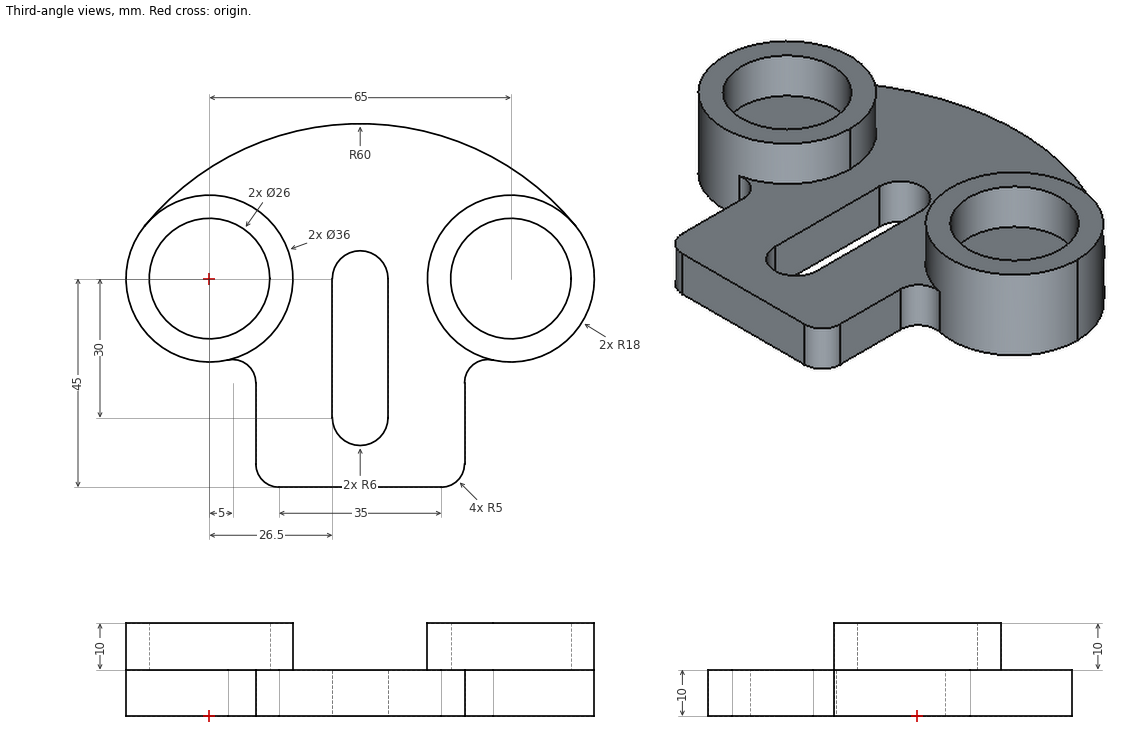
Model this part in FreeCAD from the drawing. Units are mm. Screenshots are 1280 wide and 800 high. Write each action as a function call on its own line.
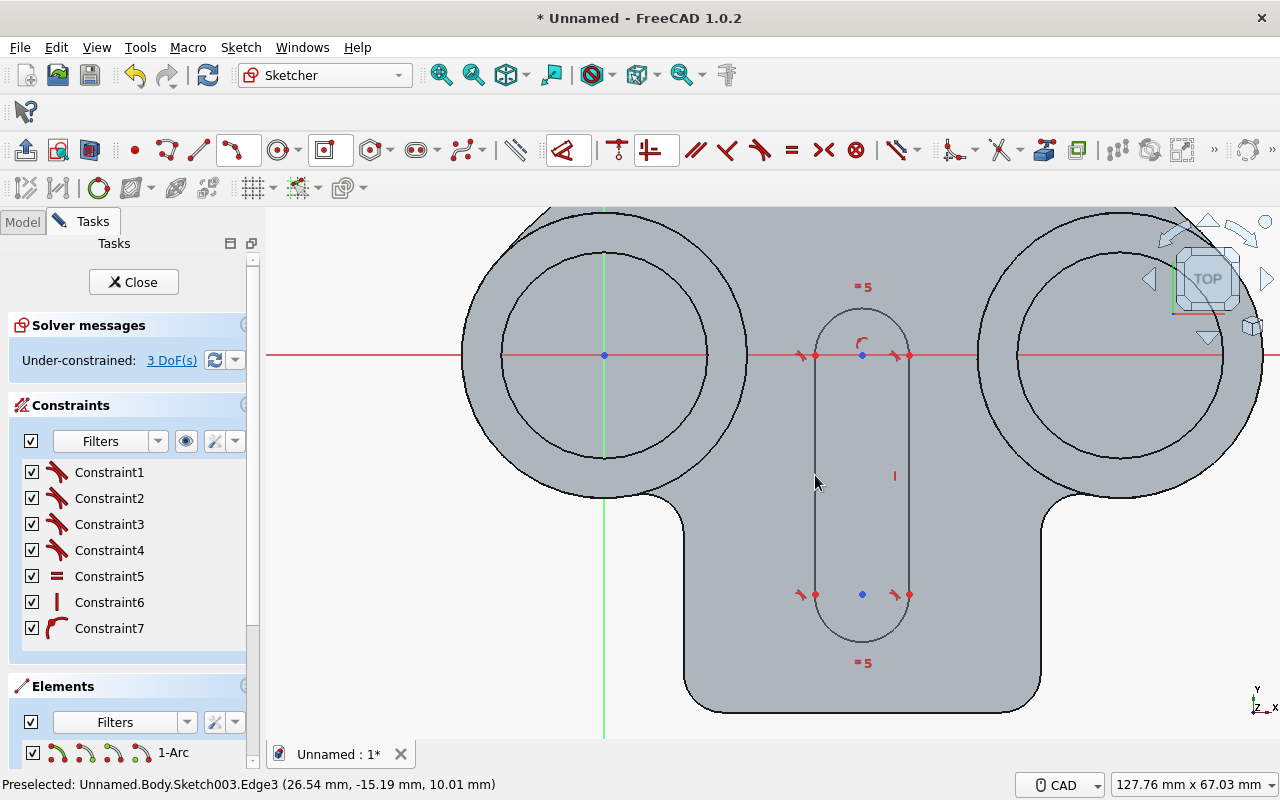
click(834, 633)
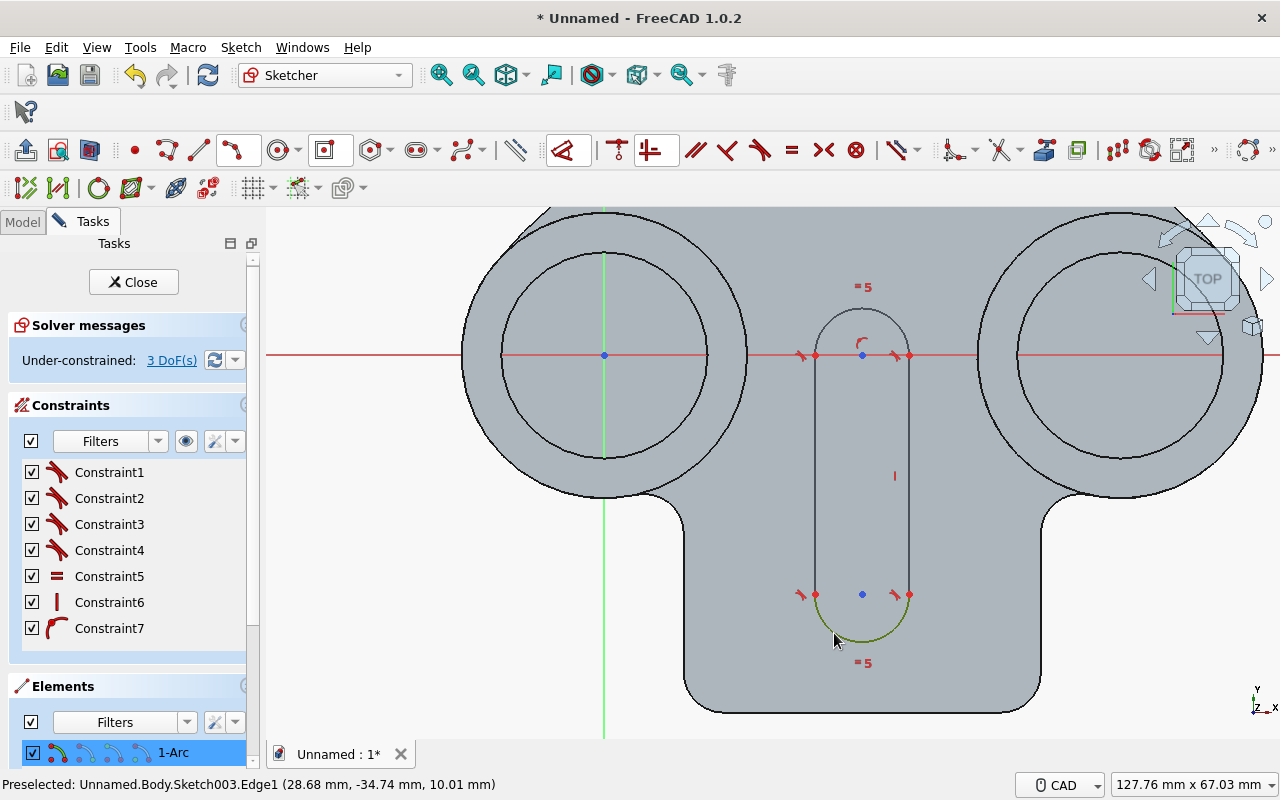
key(k)
key(r)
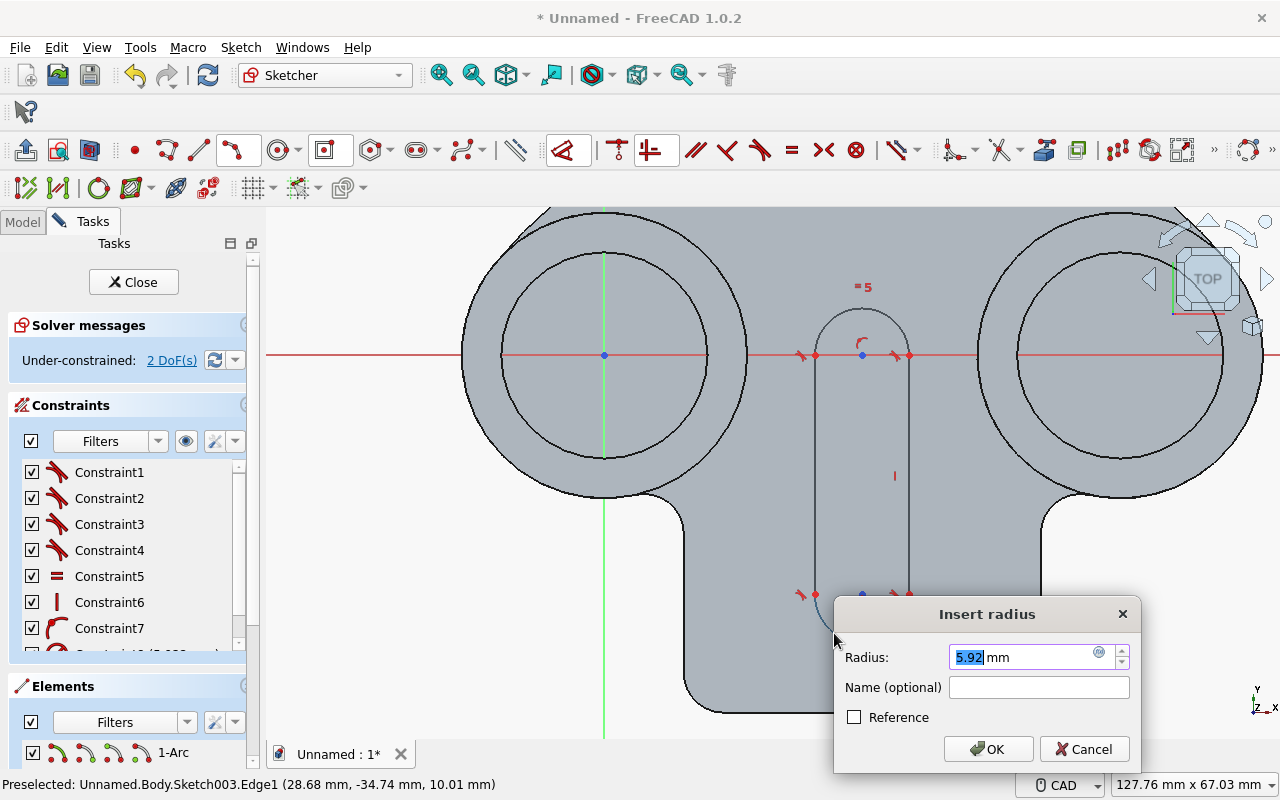
text(6)
key(Return)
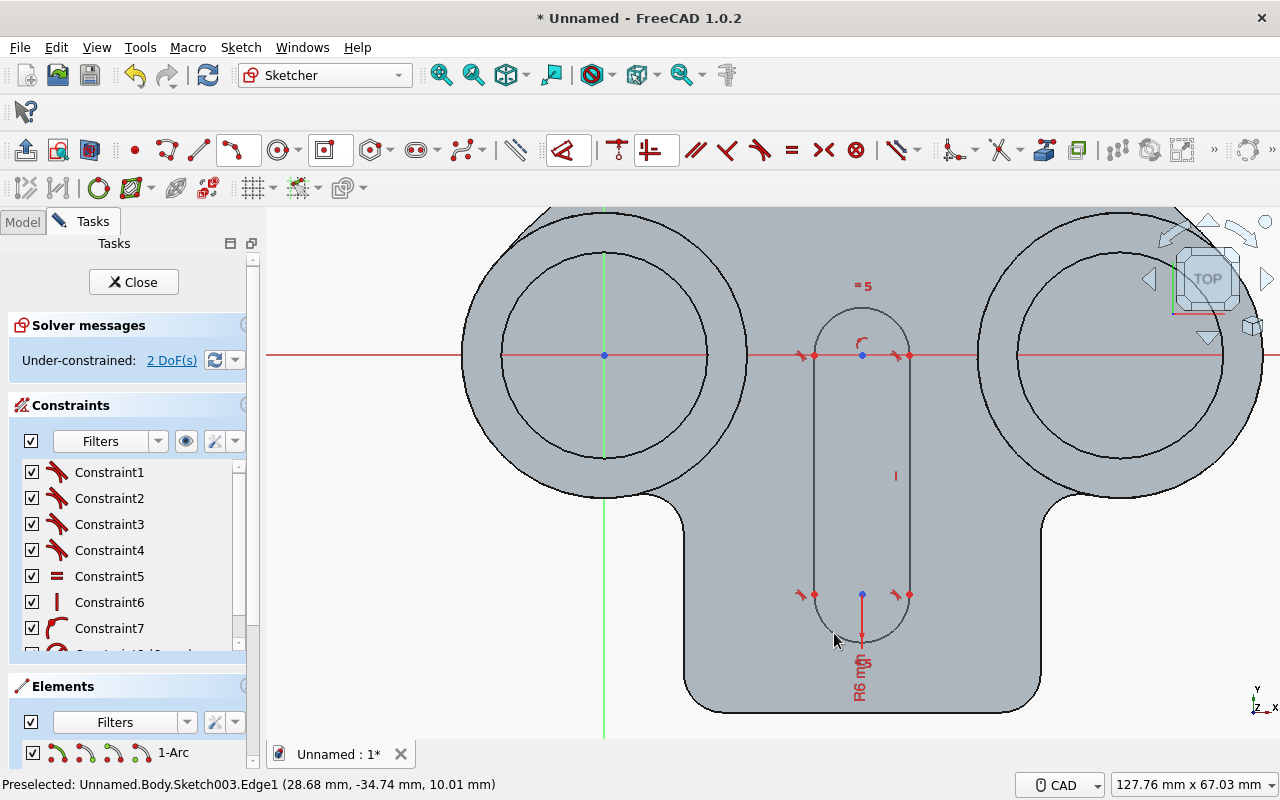
click(814, 523)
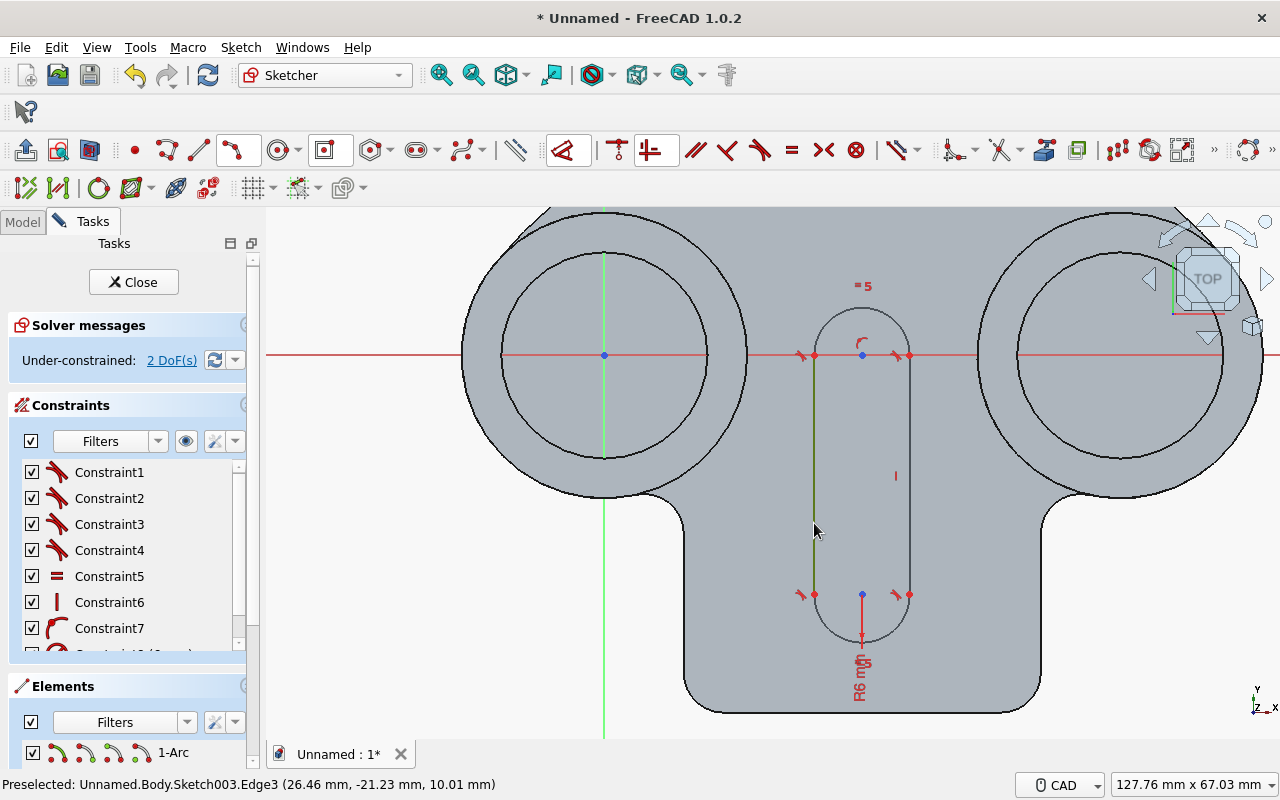
click(586, 150)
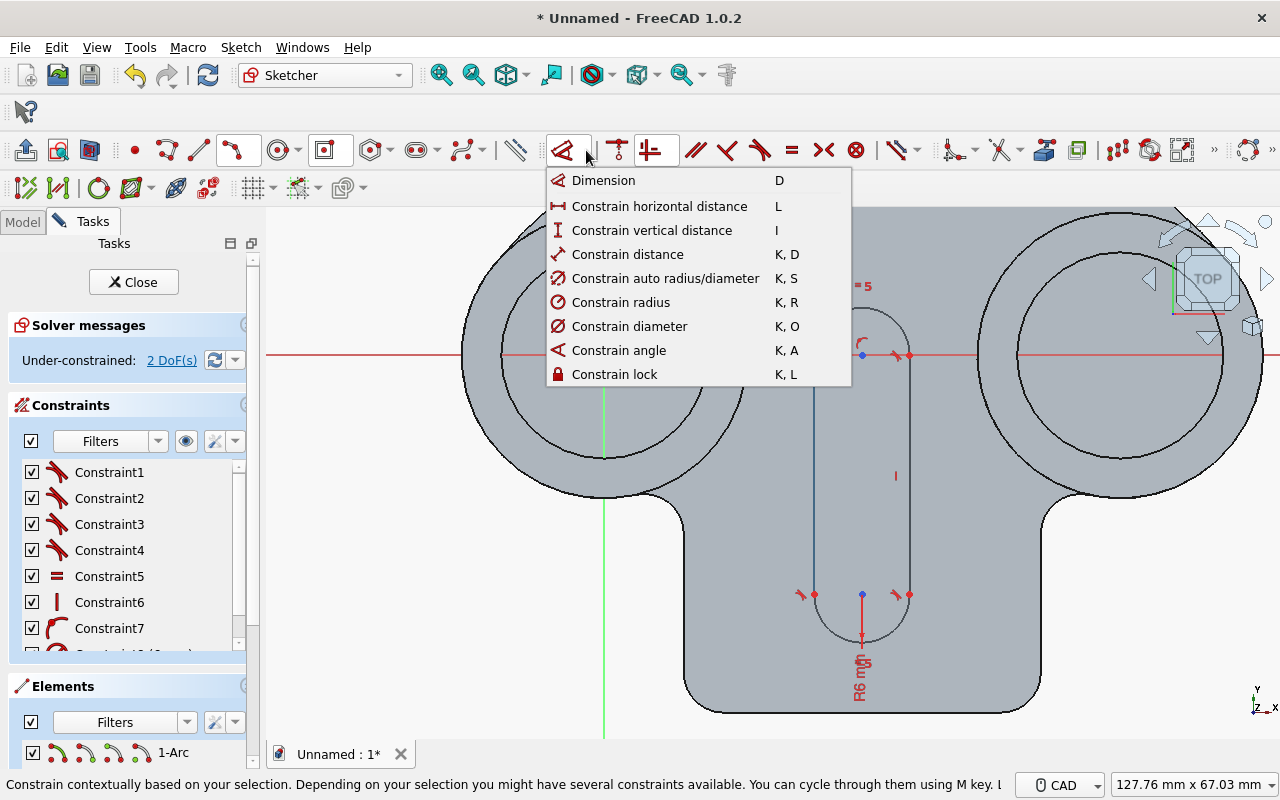
click(699, 230)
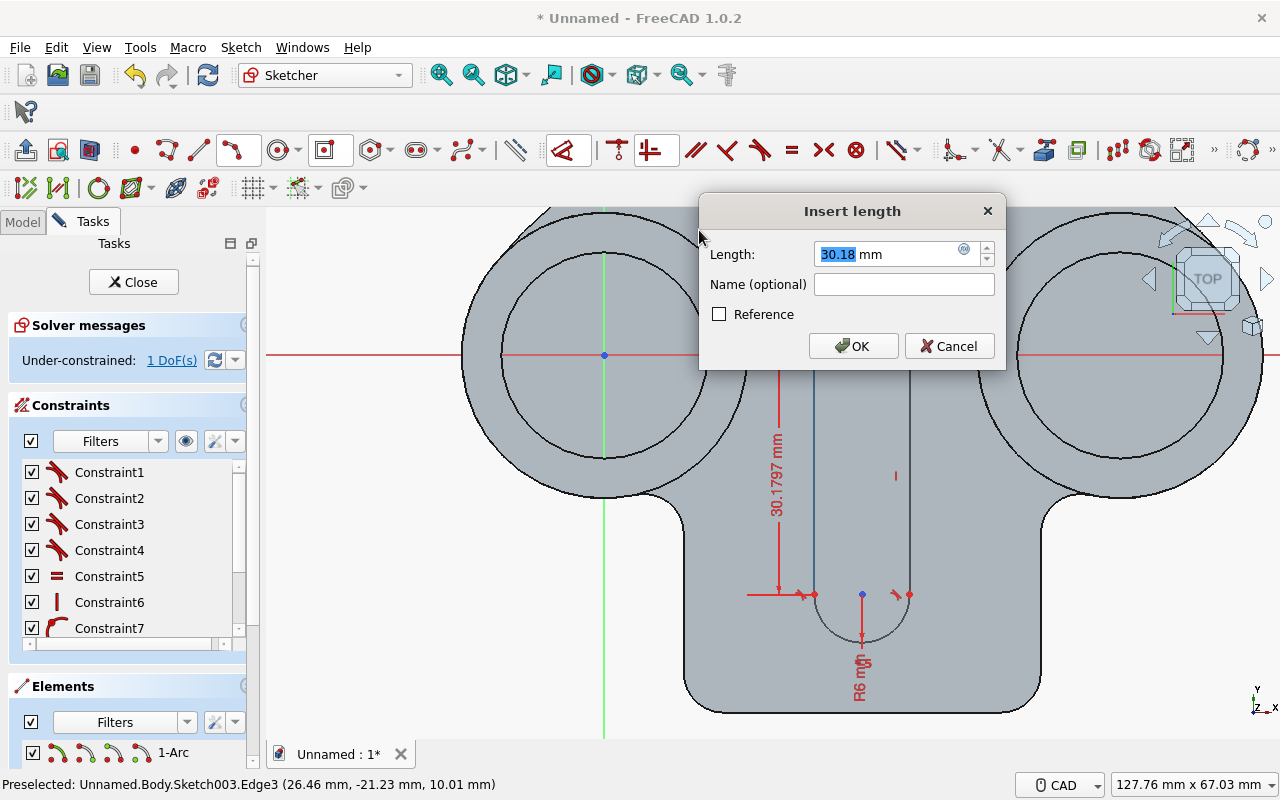
text(30)
key(Return)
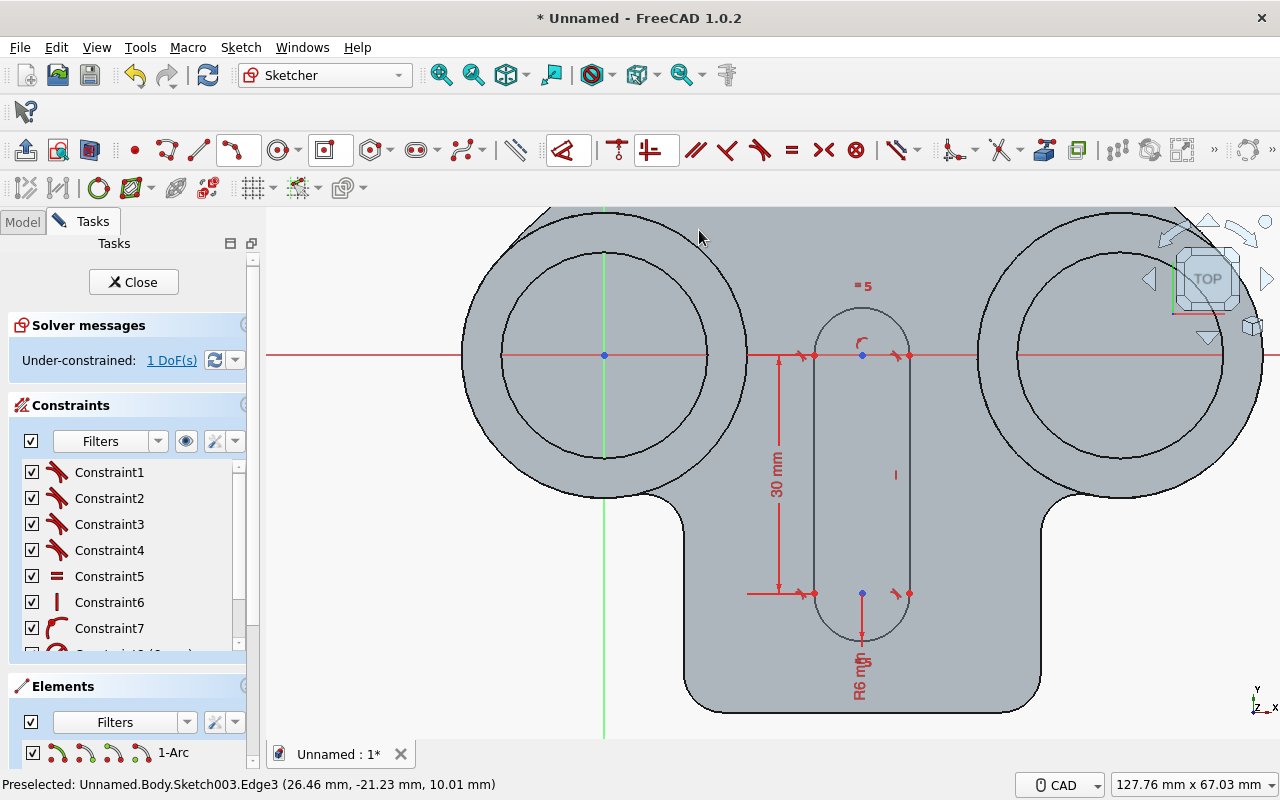
click(814, 594)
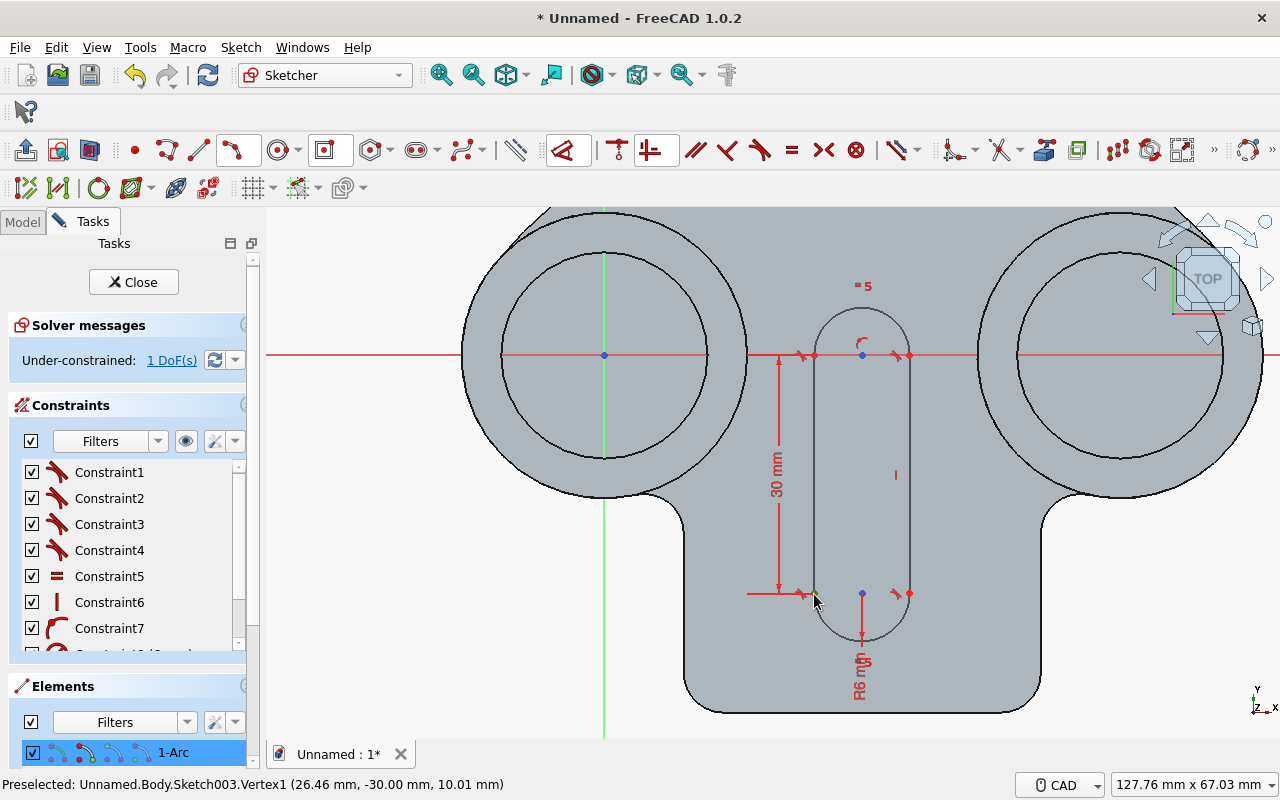
click(586, 150)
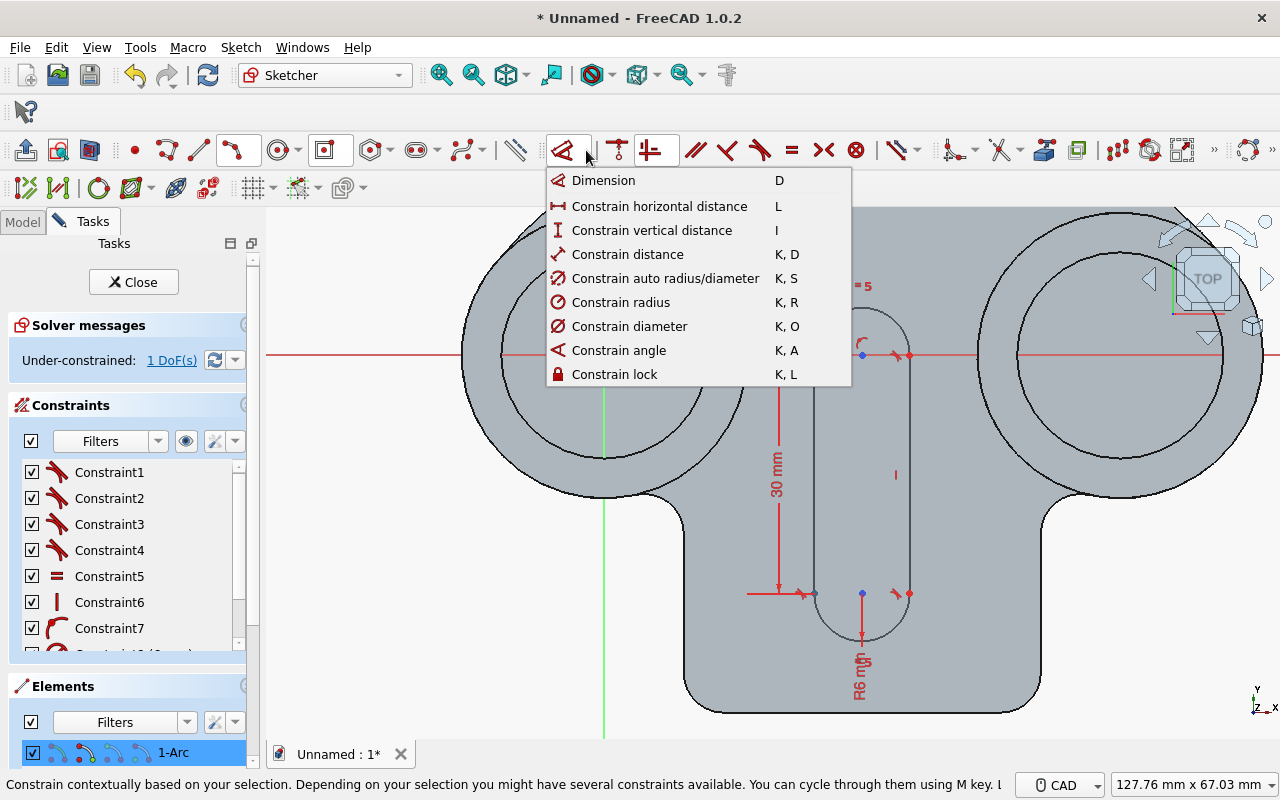
click(699, 206)